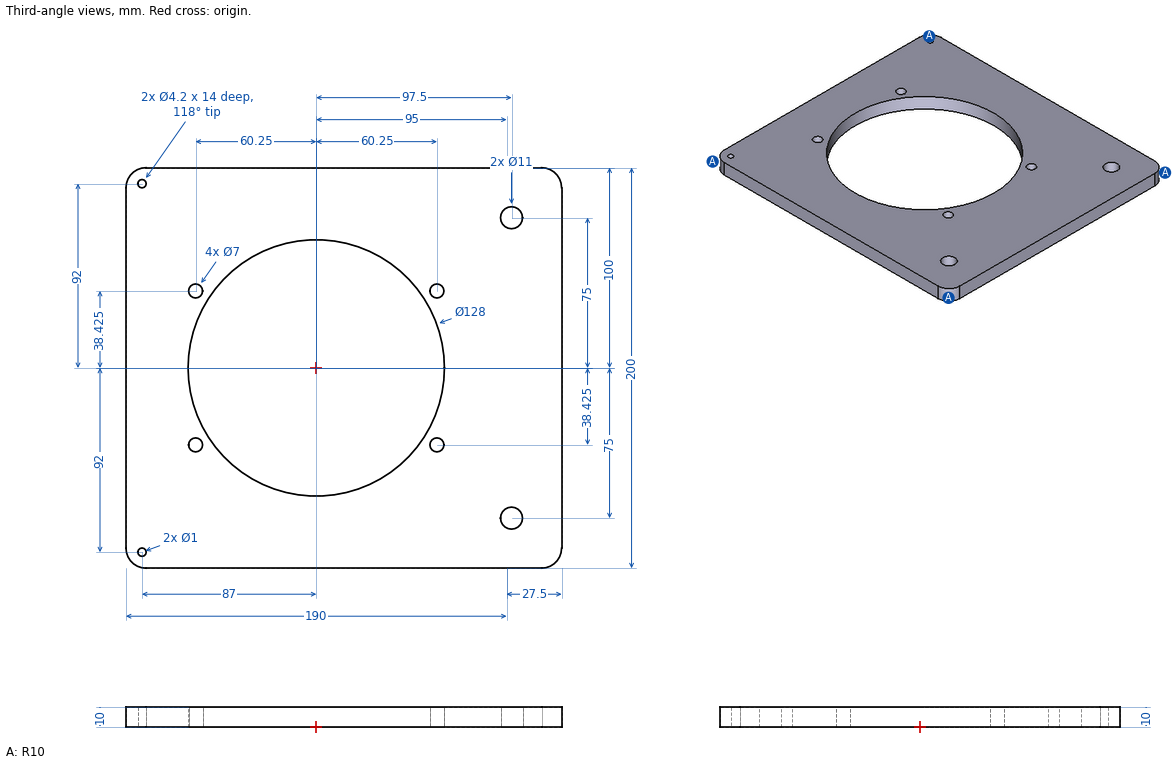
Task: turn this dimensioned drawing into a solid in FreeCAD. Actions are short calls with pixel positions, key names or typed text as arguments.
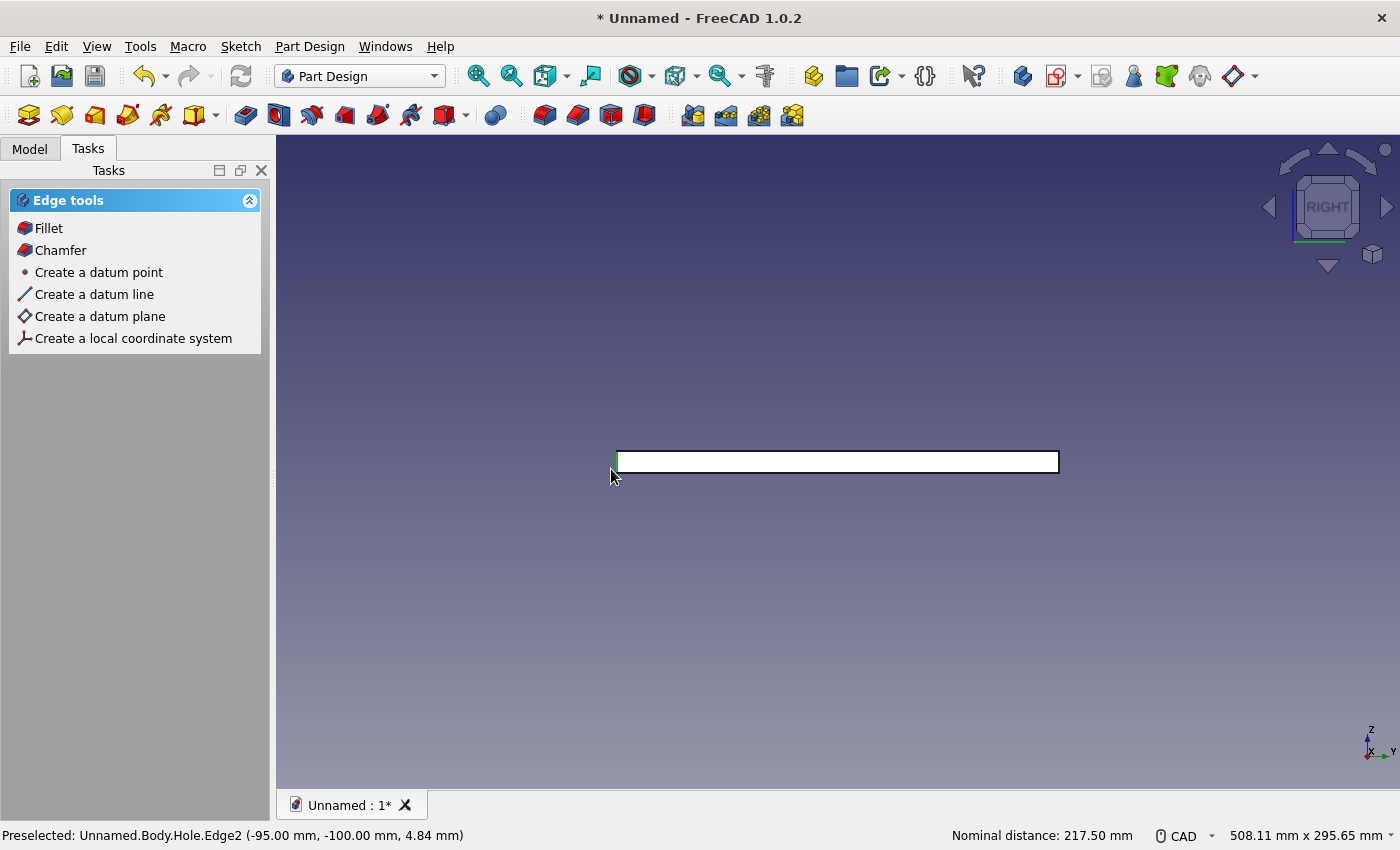
click(1059, 461, ctrl)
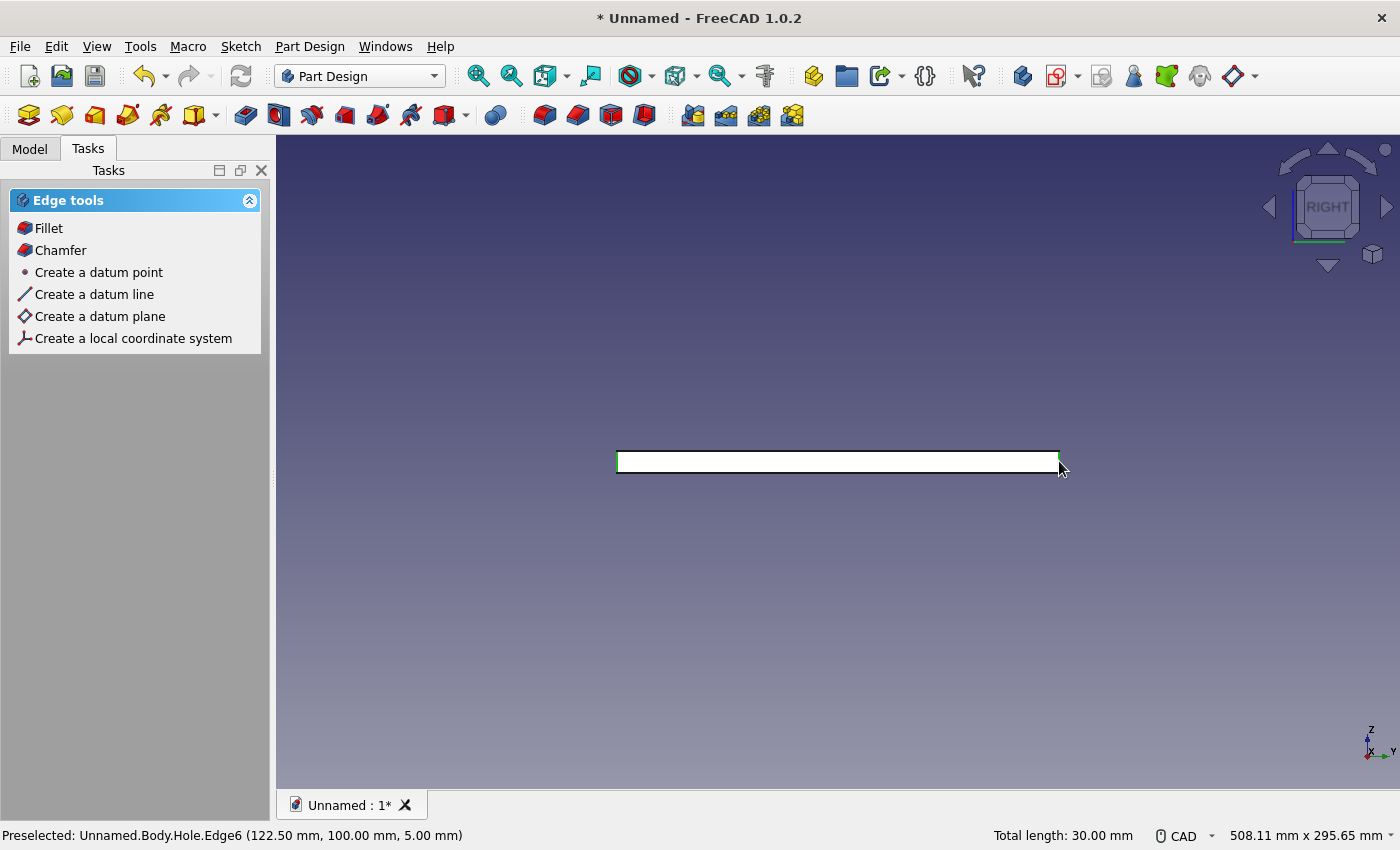
key(5)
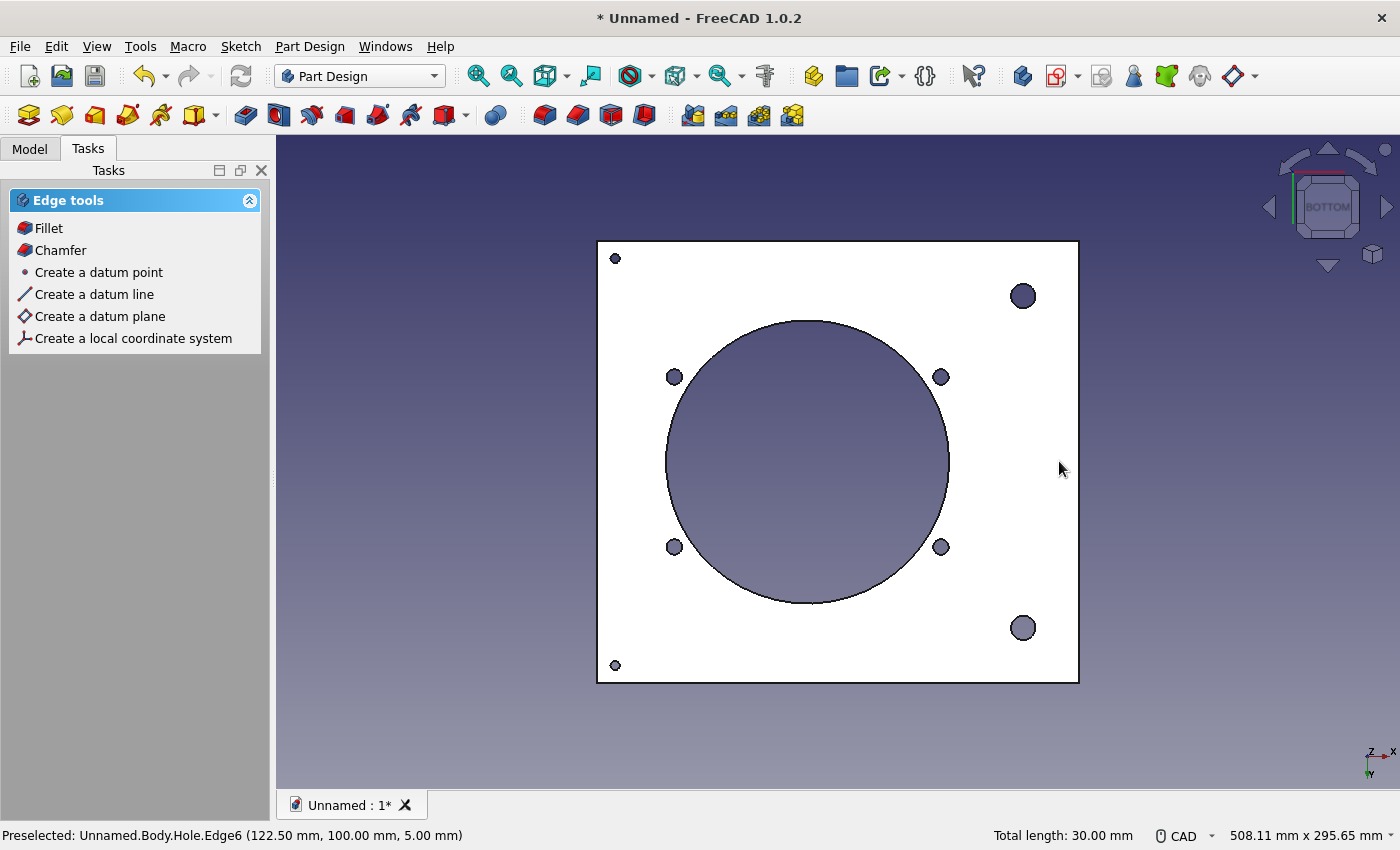
key(4)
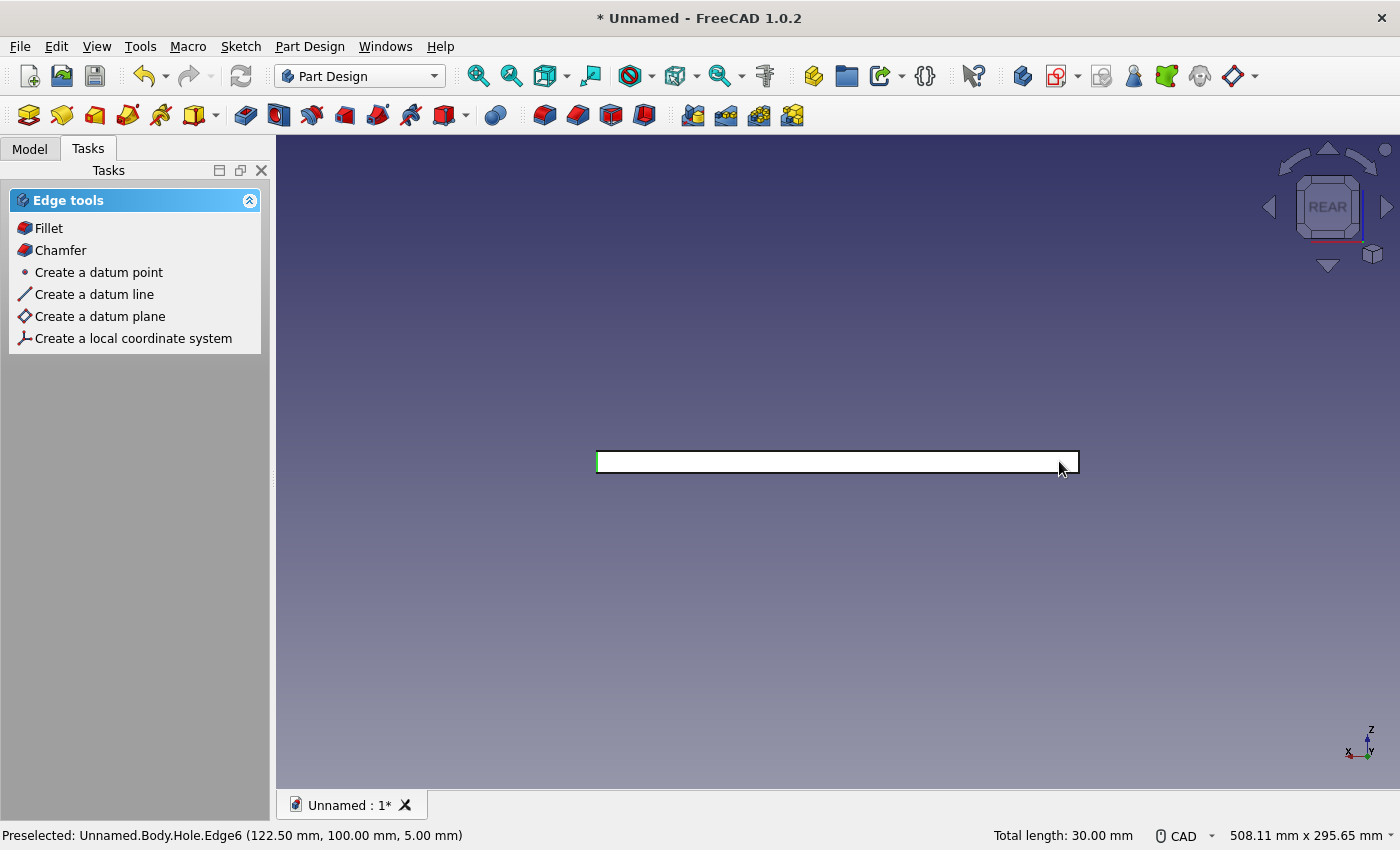
key(v)
key(f)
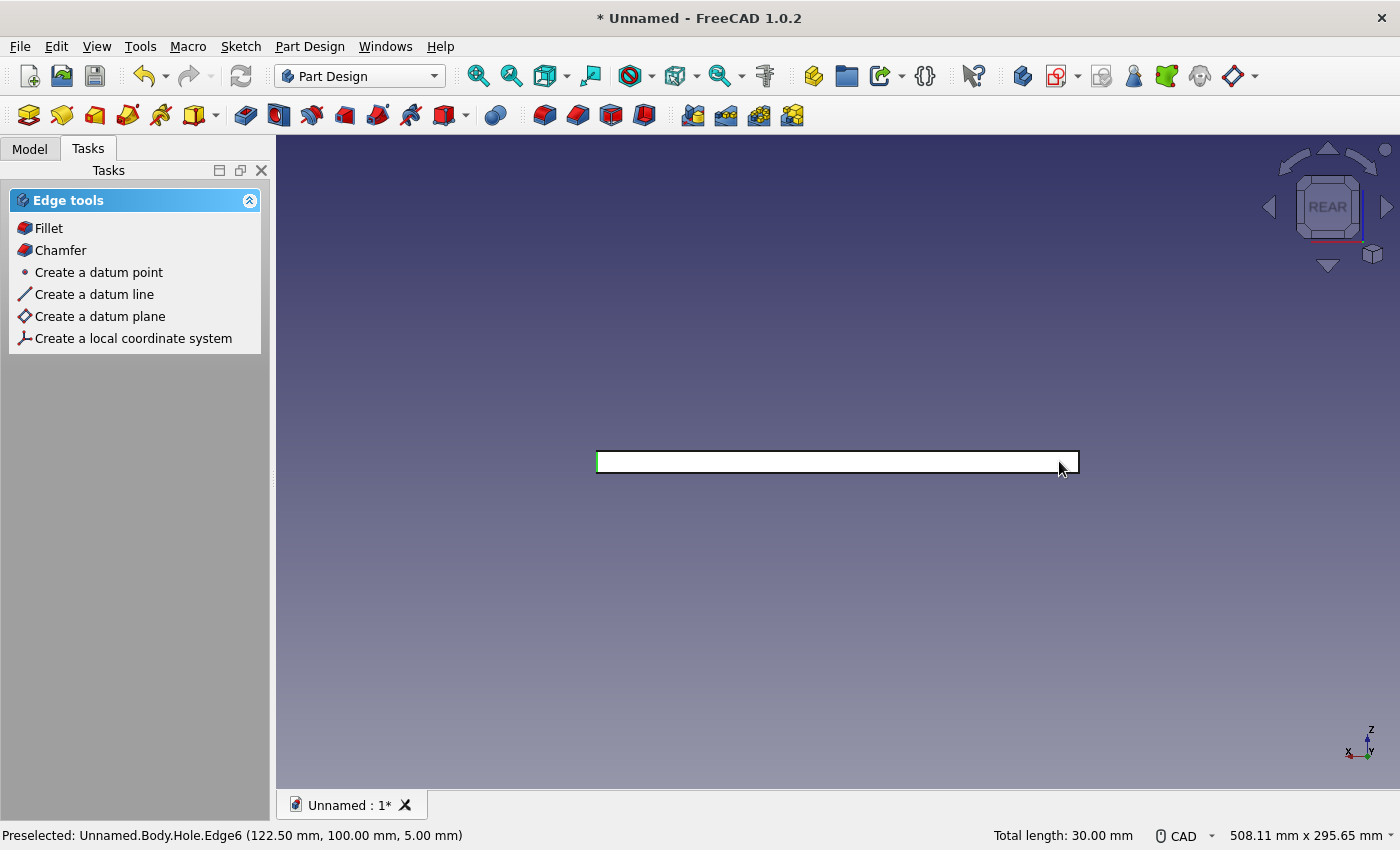
click(1079, 461, ctrl)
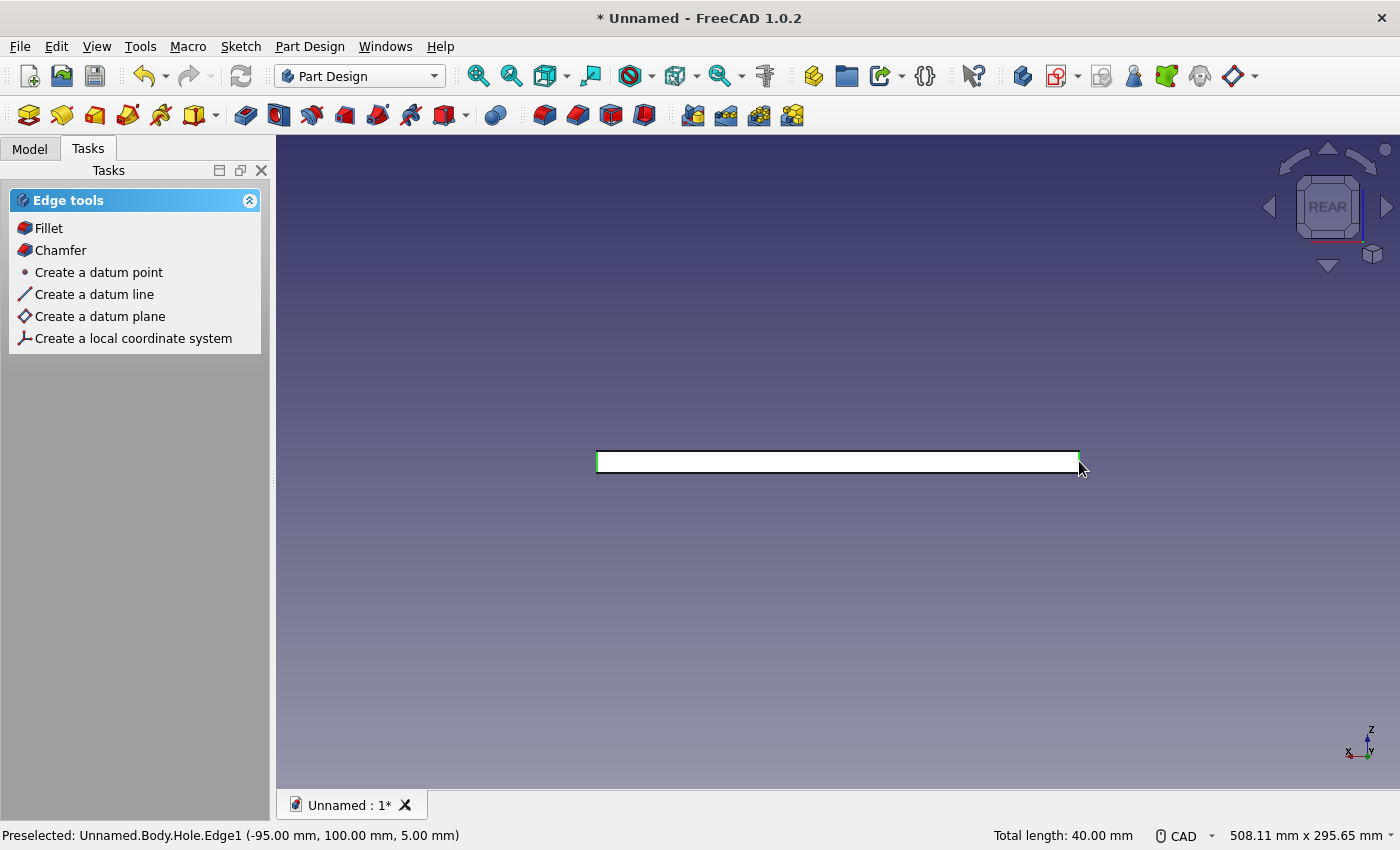
click(545, 116)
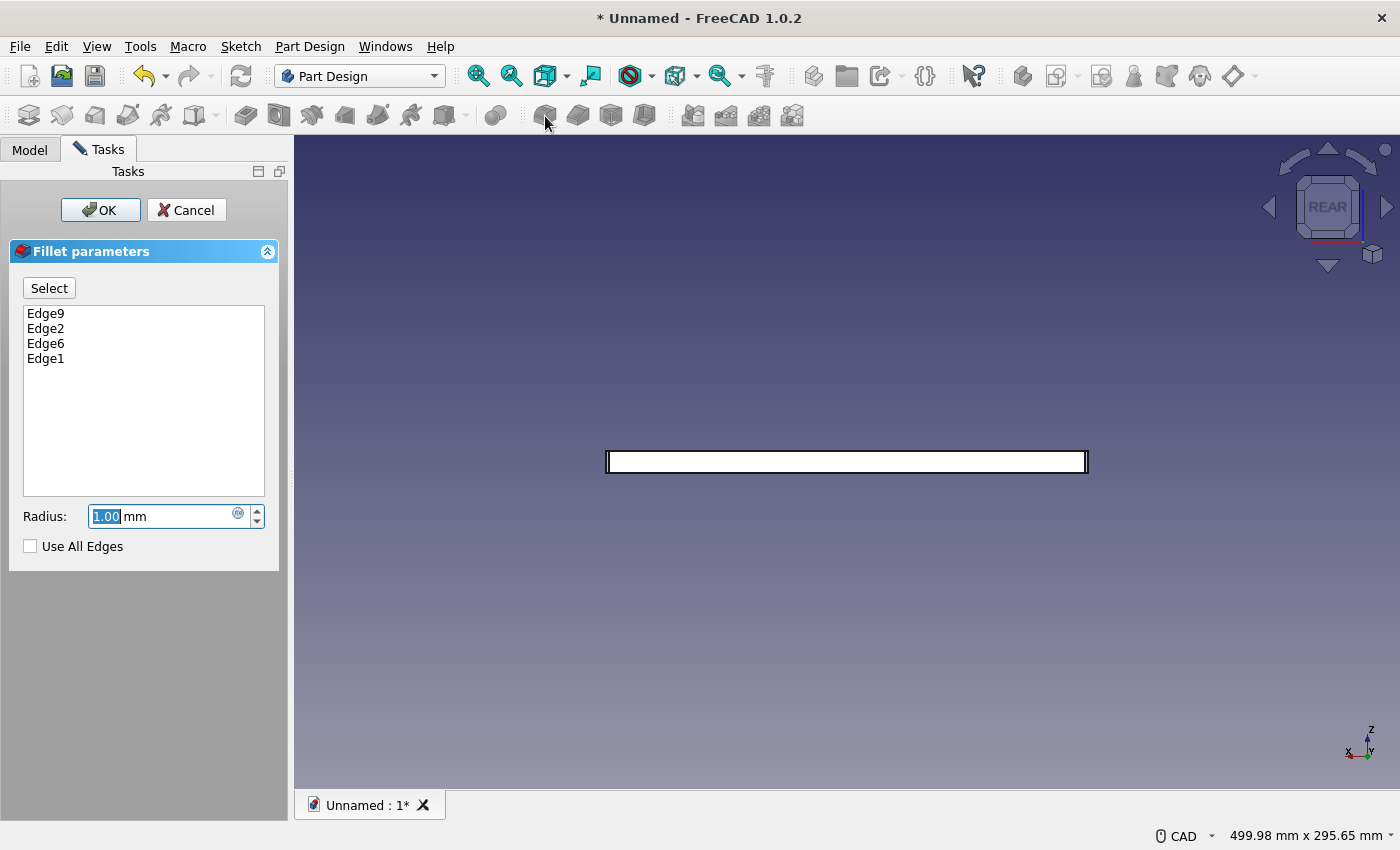
text(10)
key(Tab)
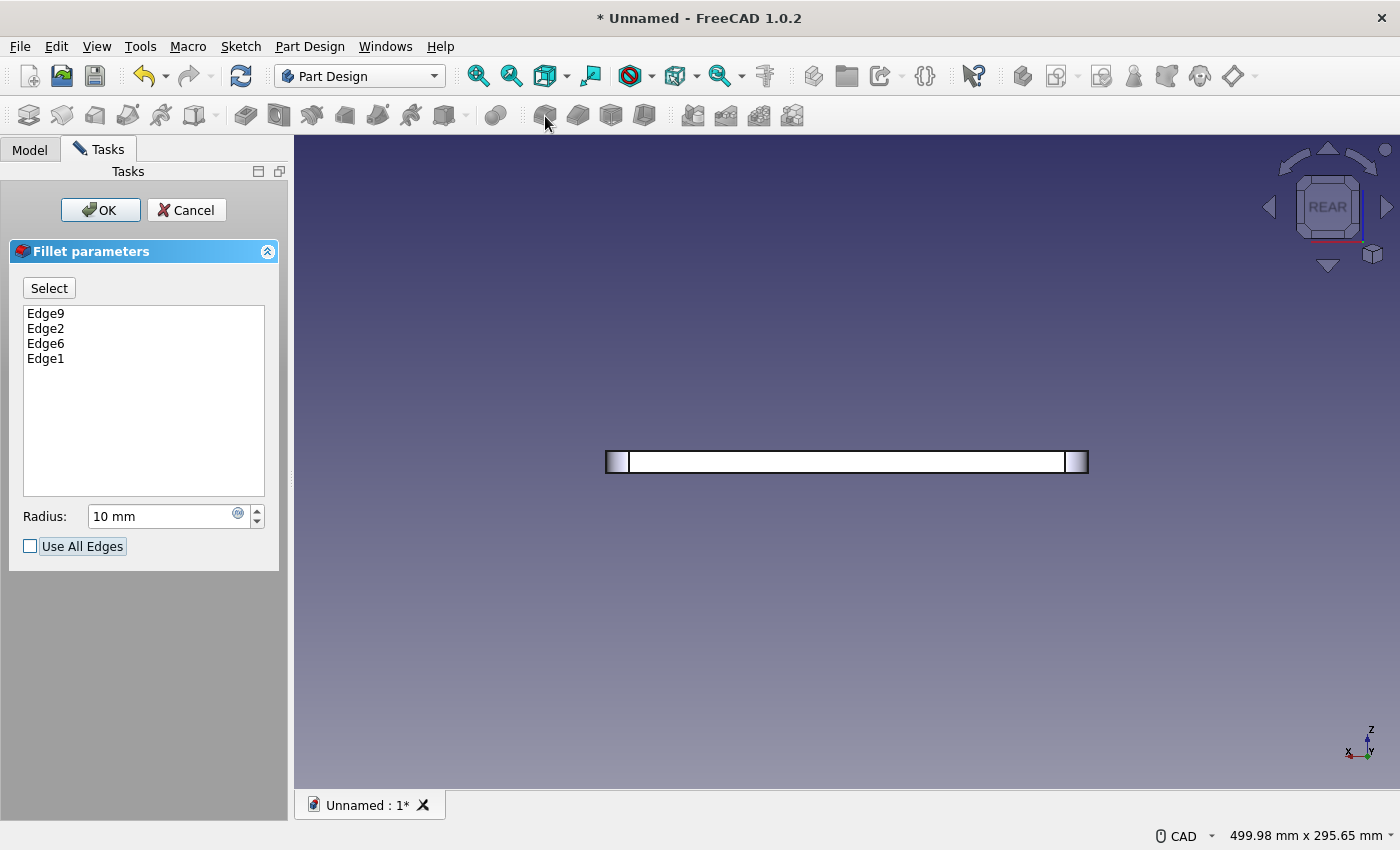
click(101, 210)